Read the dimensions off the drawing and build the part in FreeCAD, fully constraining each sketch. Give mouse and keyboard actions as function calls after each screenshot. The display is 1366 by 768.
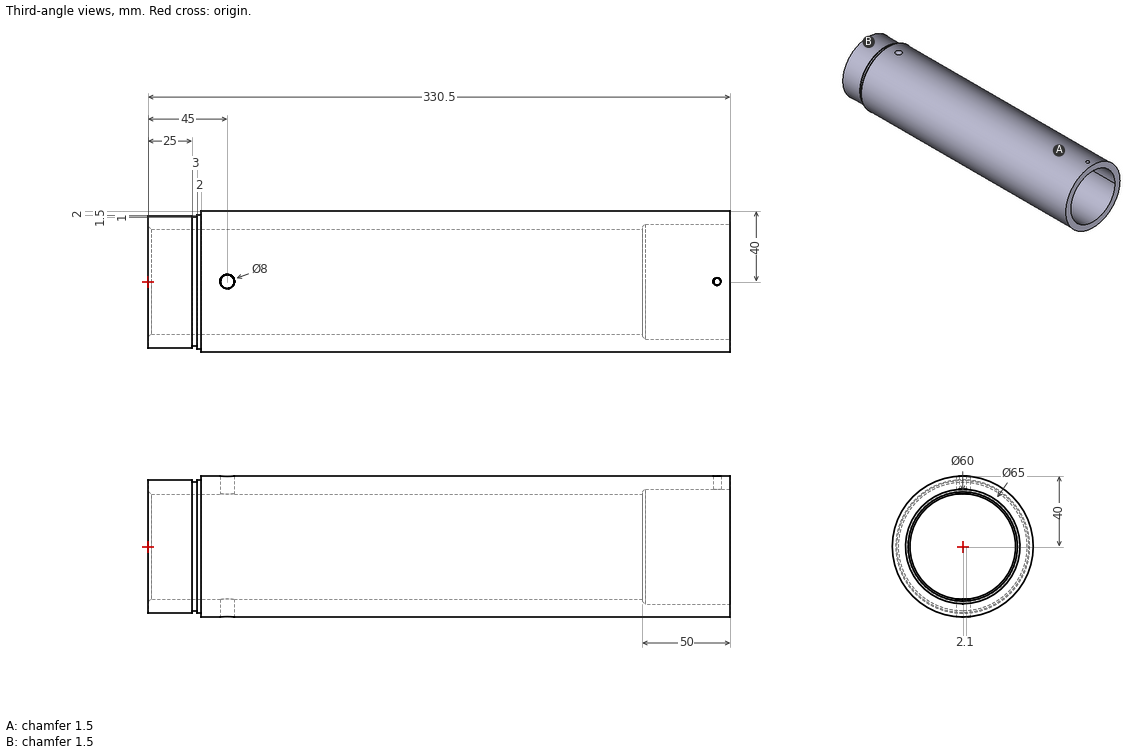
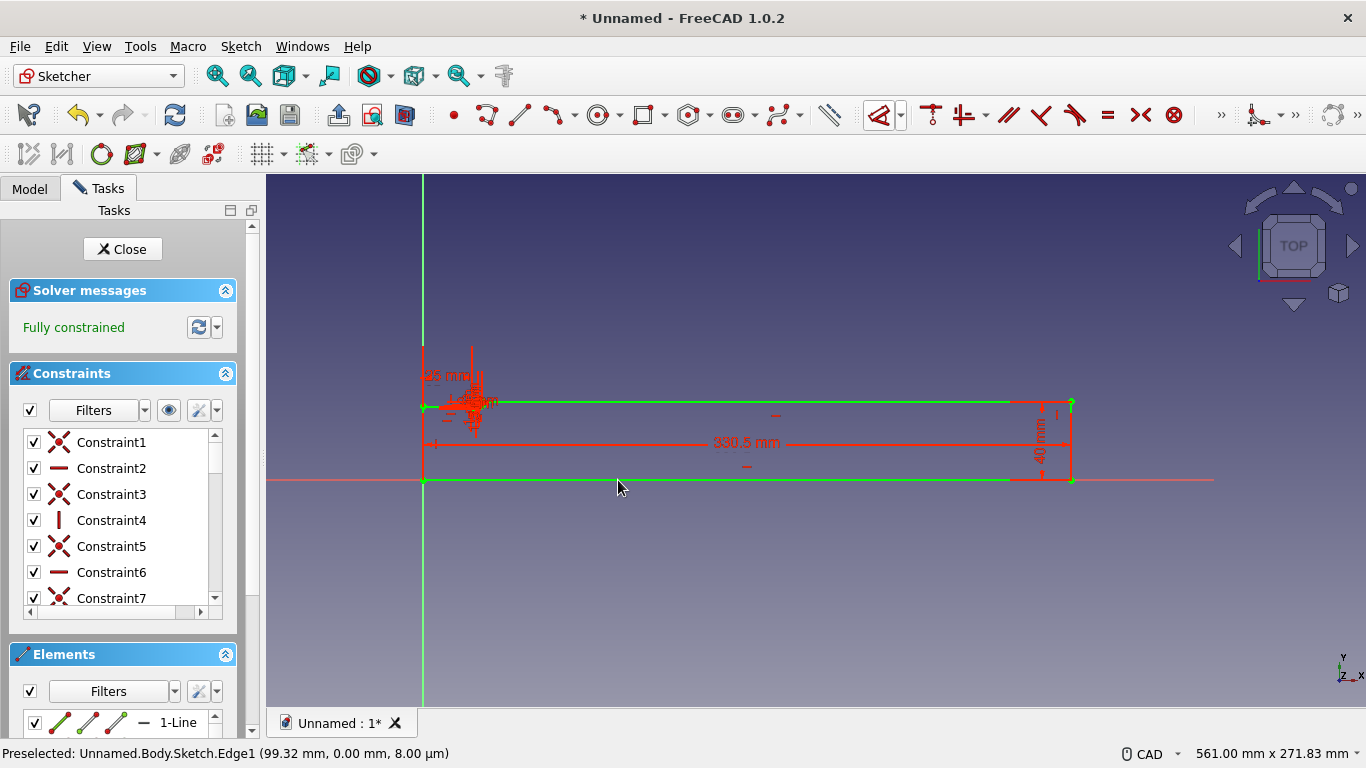
click(123, 249)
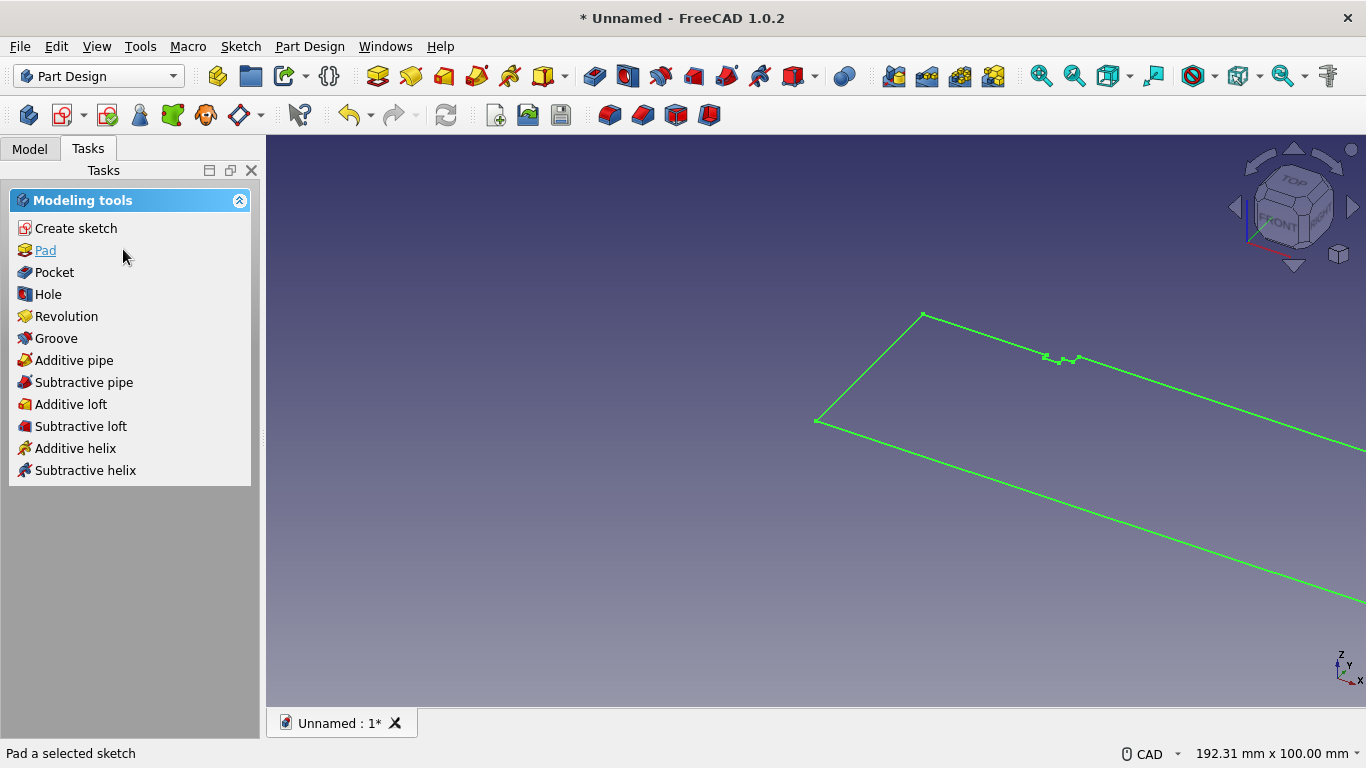
click(411, 76)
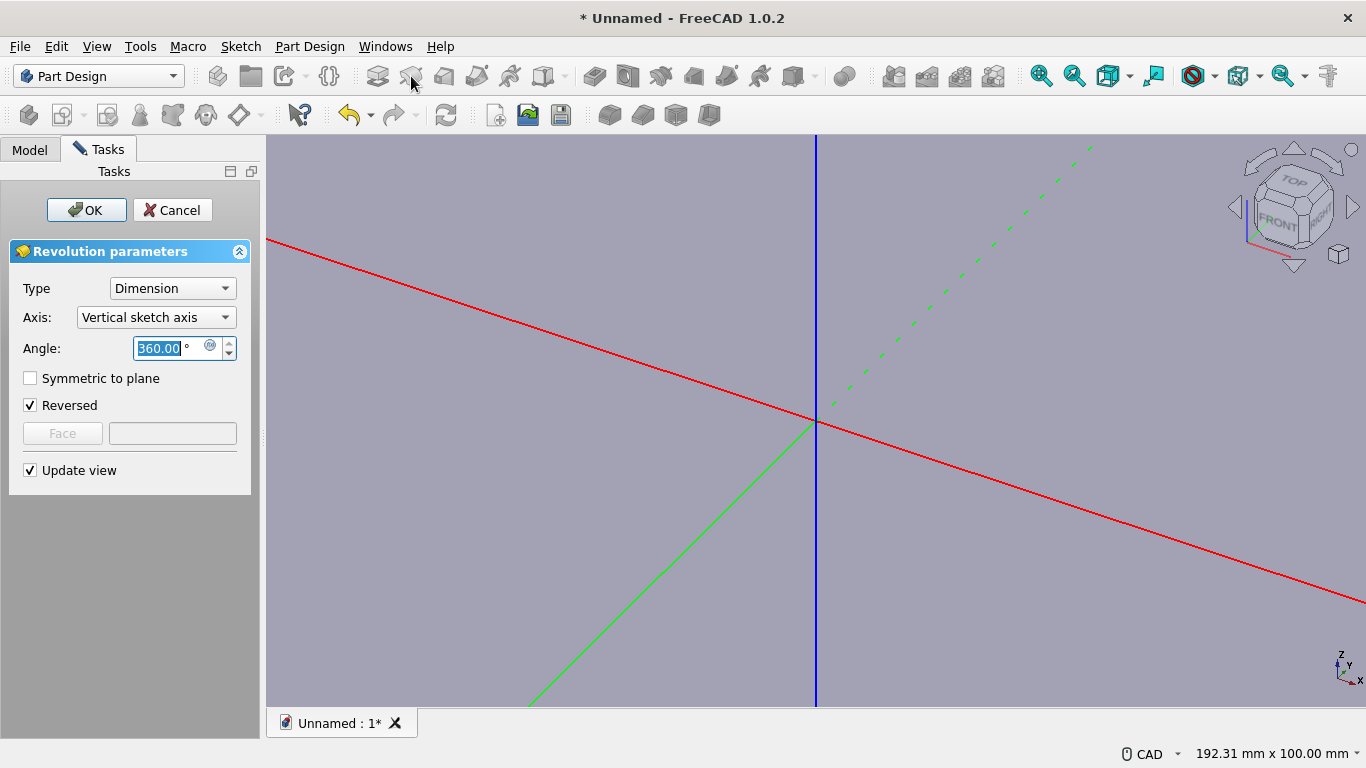
click(157, 318)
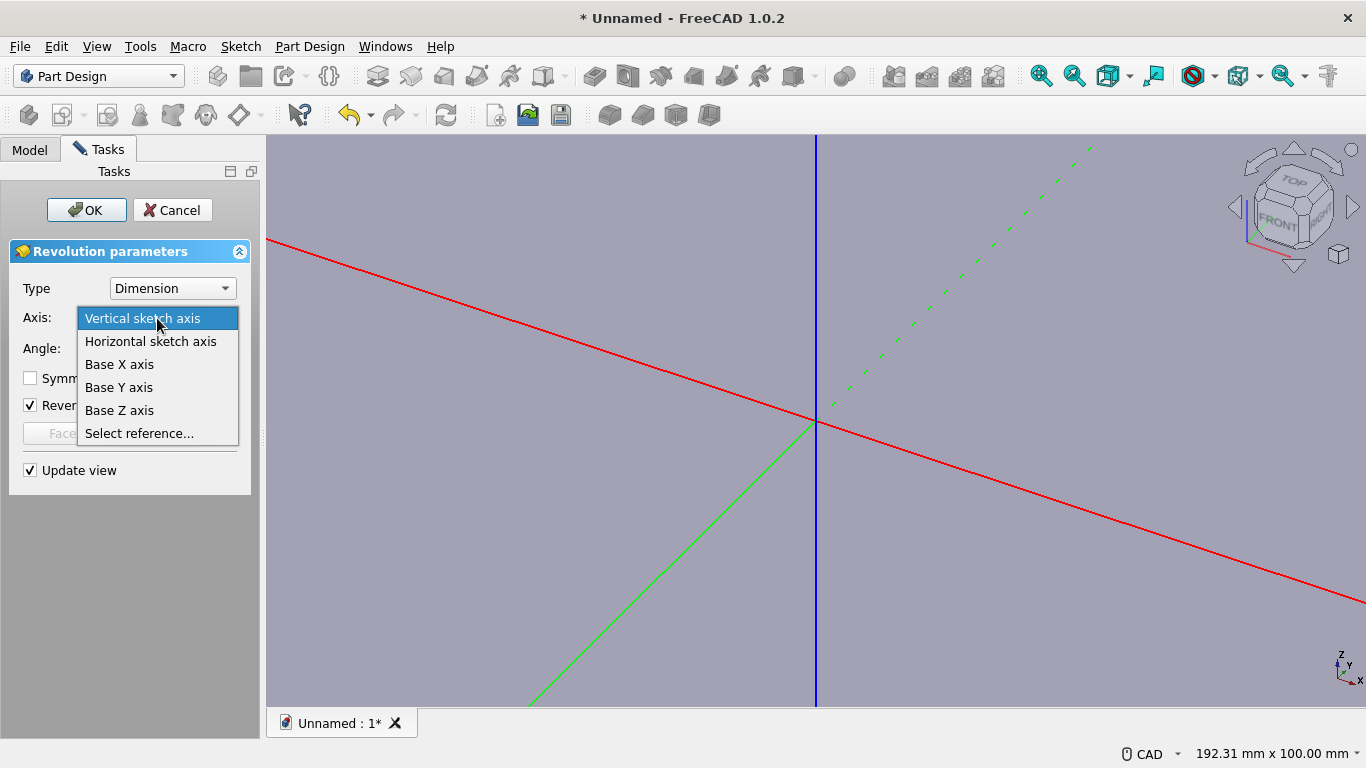
click(156, 342)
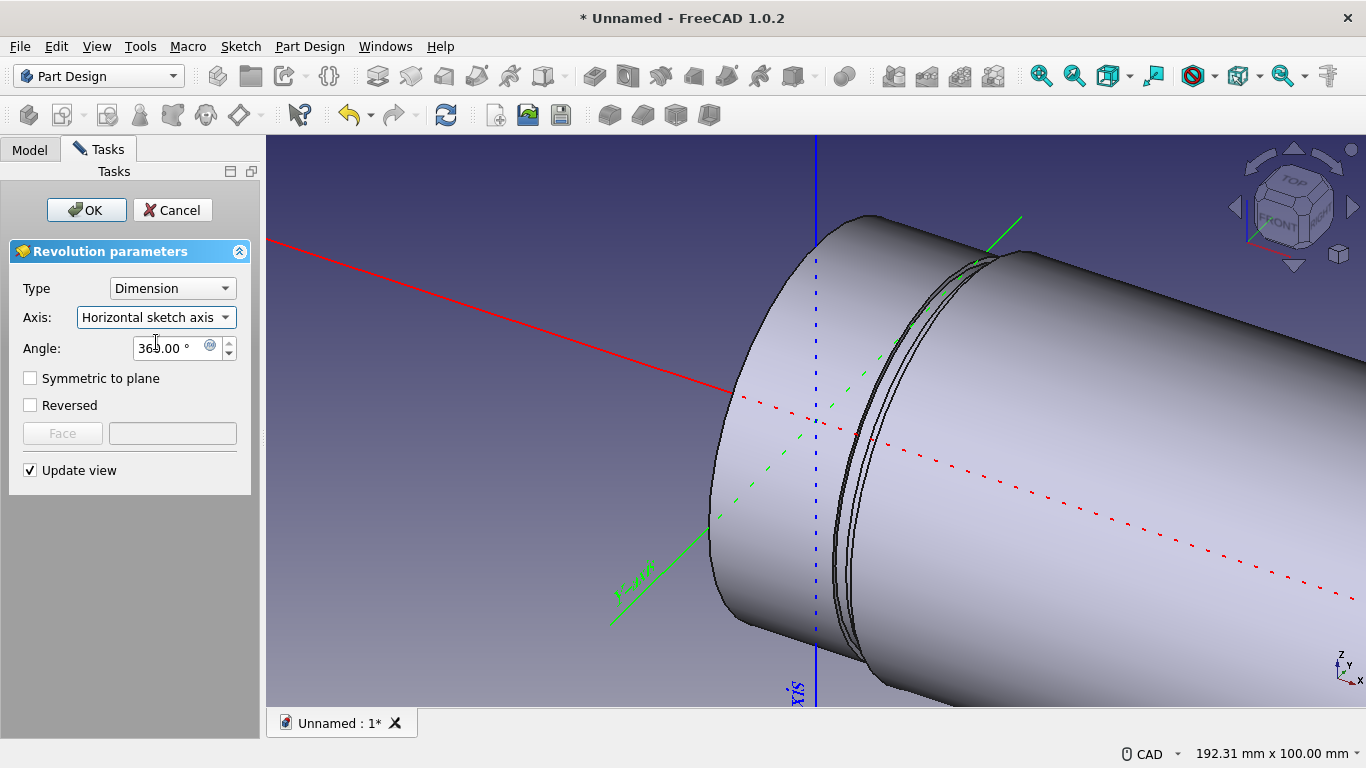
click(87, 210)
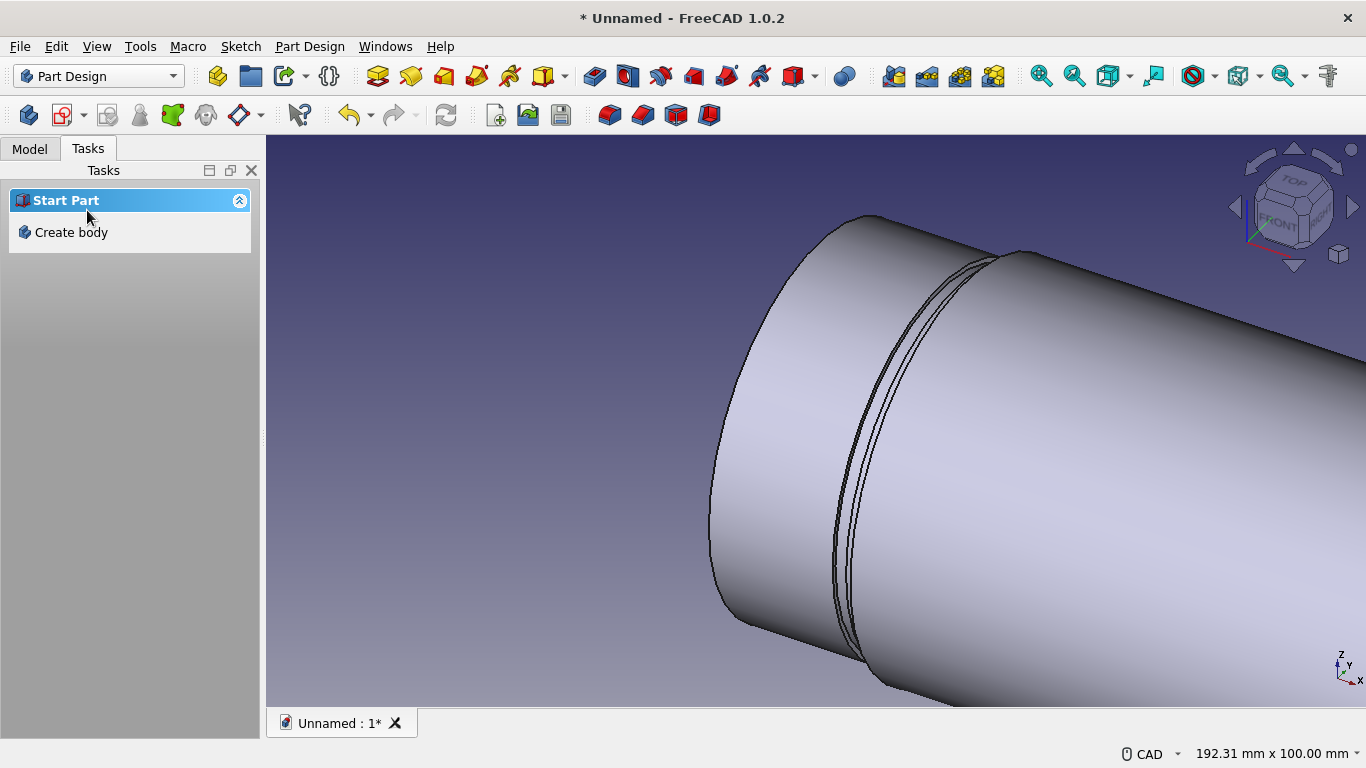
click(1042, 76)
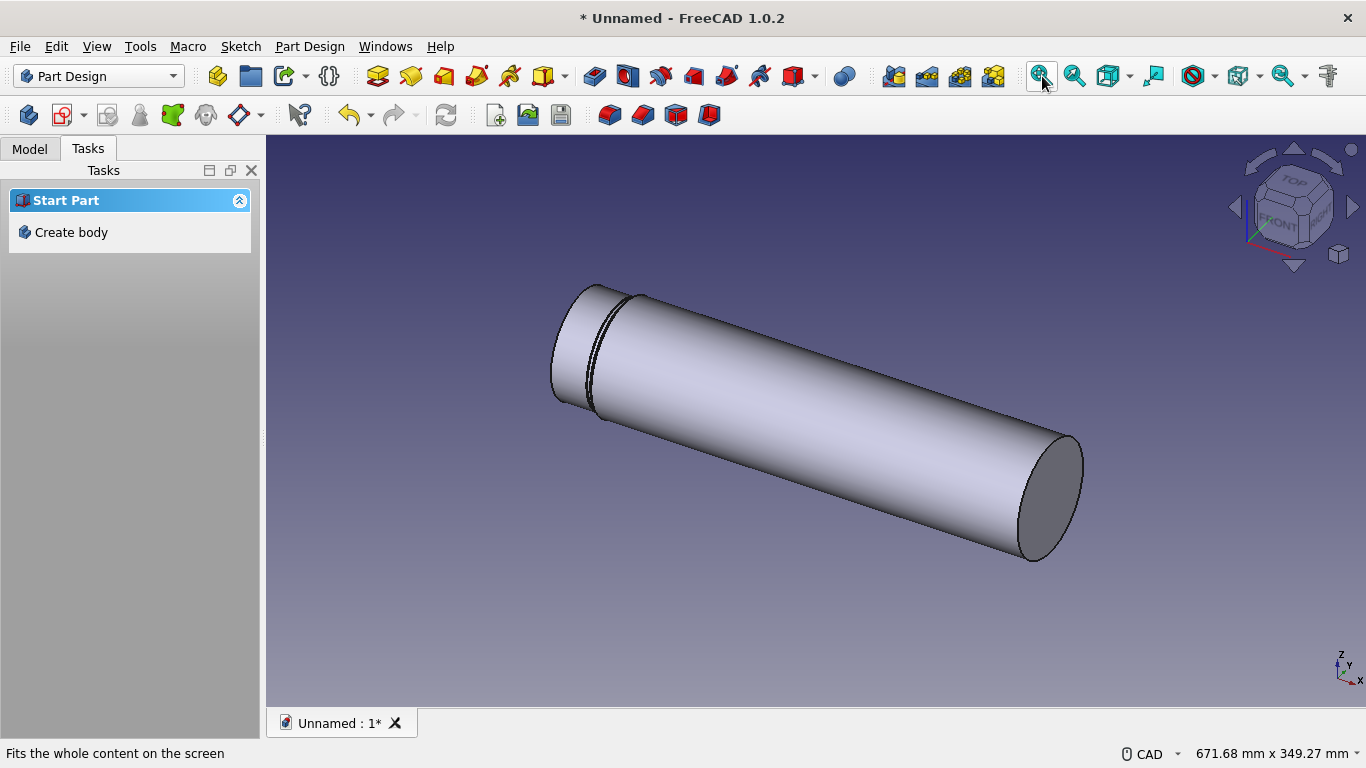
click(1050, 498)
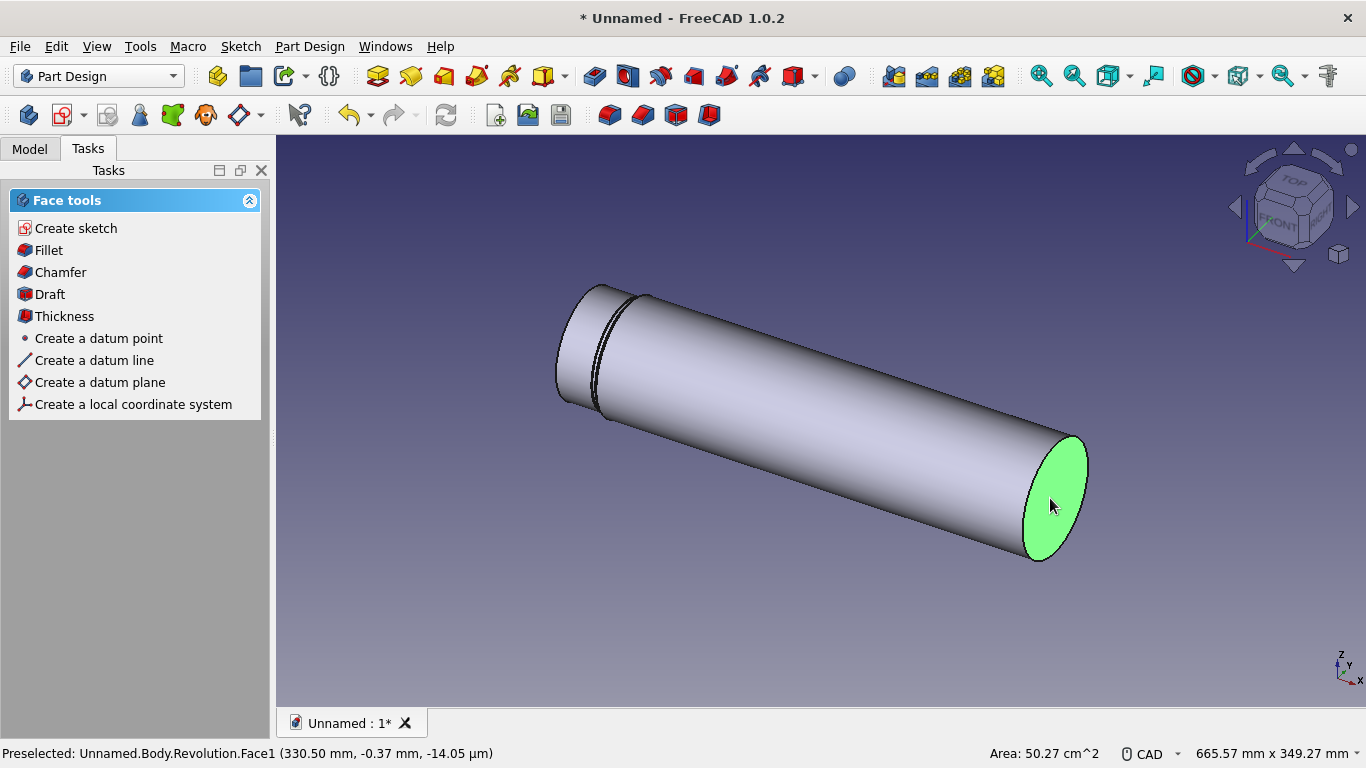
click(62, 116)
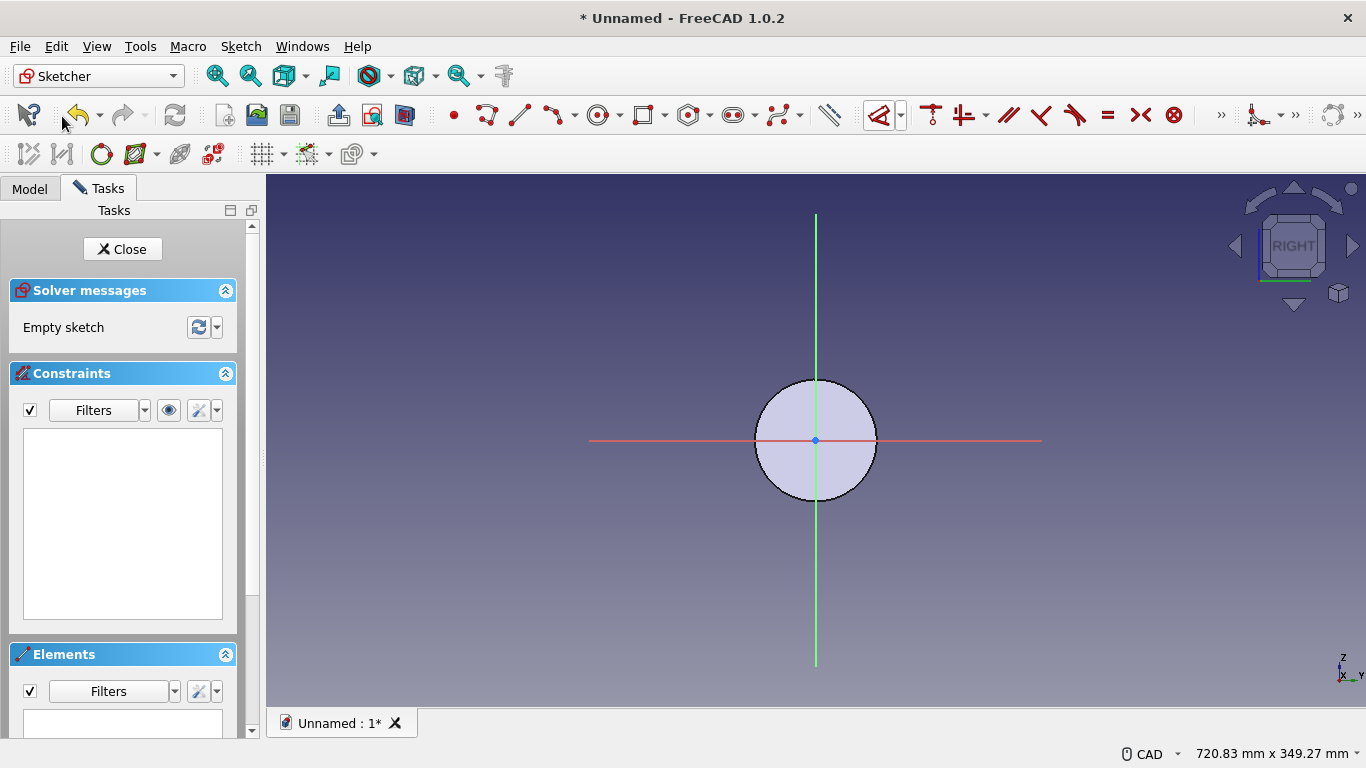
scroll(845, 440, up, 6)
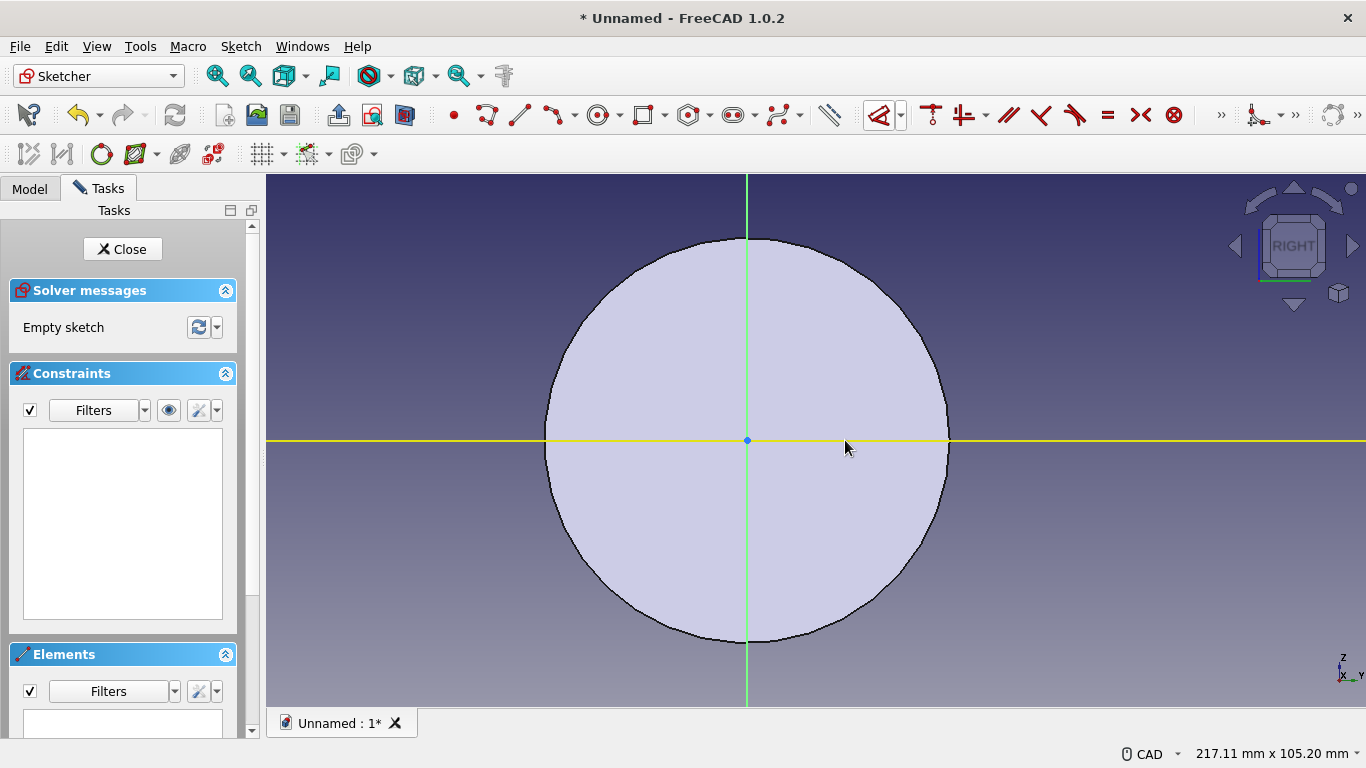
click(598, 116)